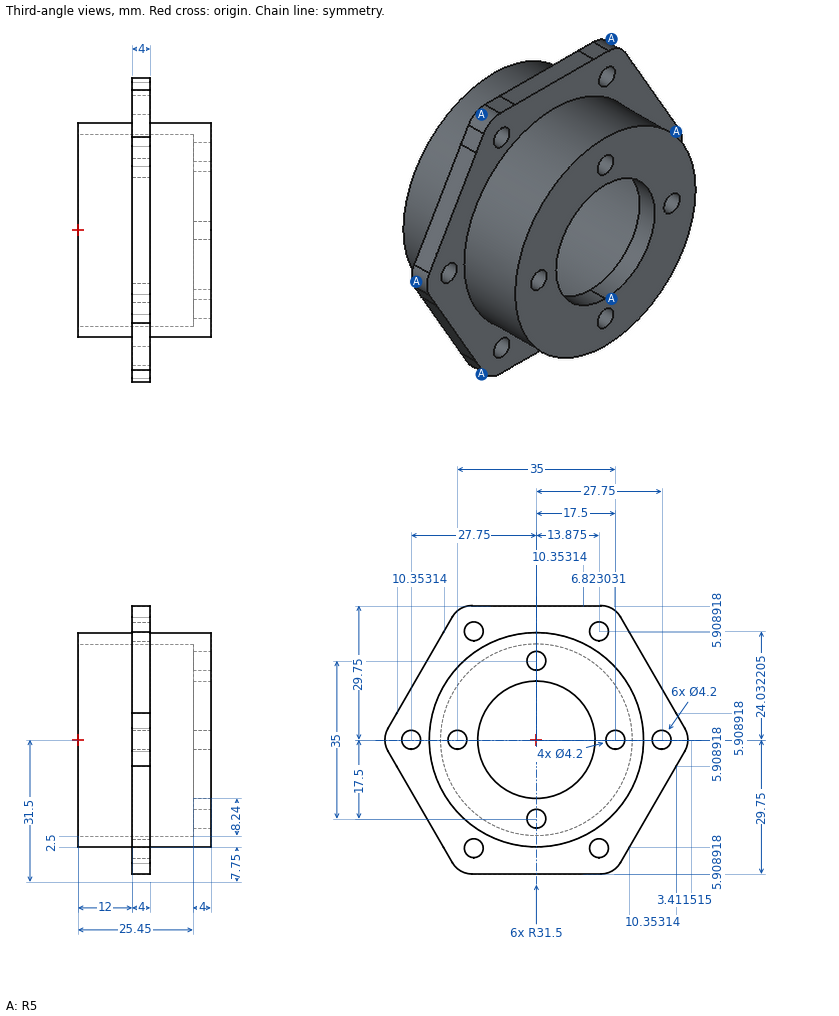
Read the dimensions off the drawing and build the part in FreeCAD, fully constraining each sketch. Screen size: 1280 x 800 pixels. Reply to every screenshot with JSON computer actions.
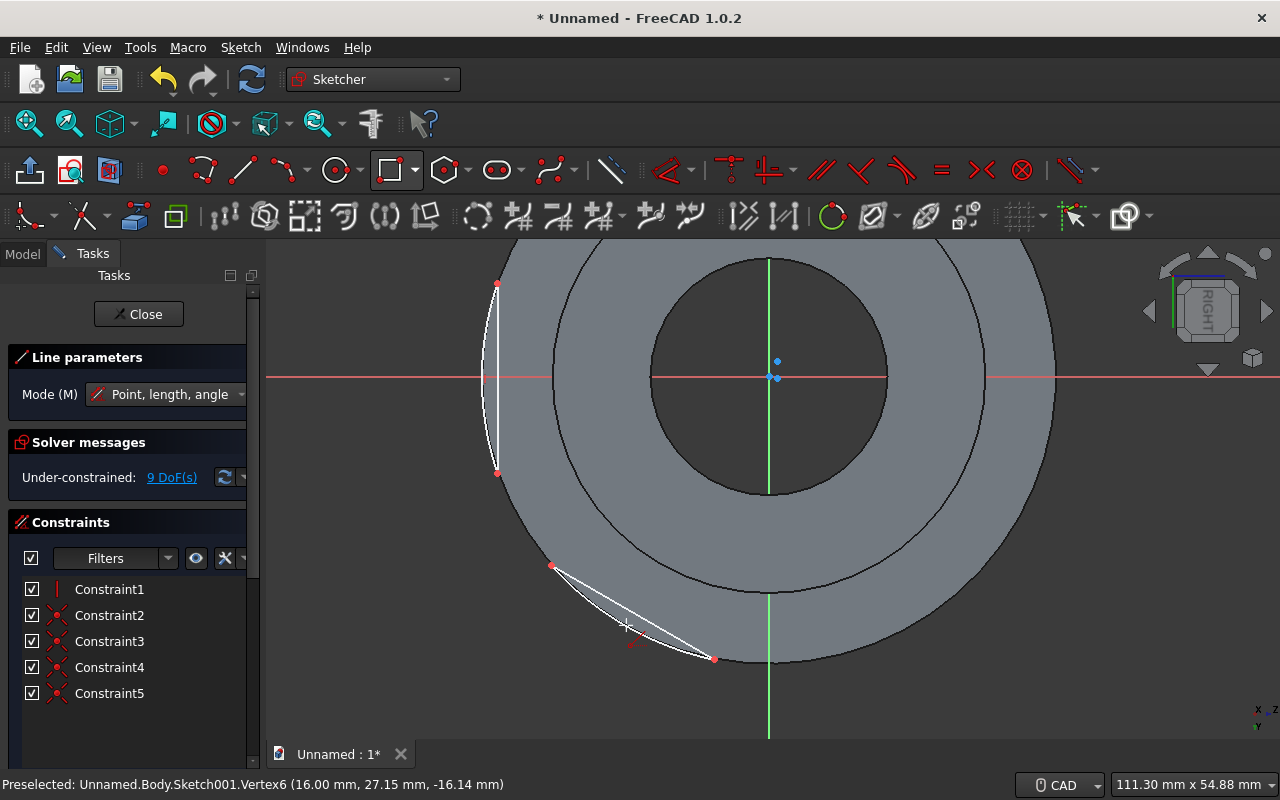
{"action": "left_click", "coordinate": [986, 564]}
{"action": "left_click", "coordinate": [823, 659]}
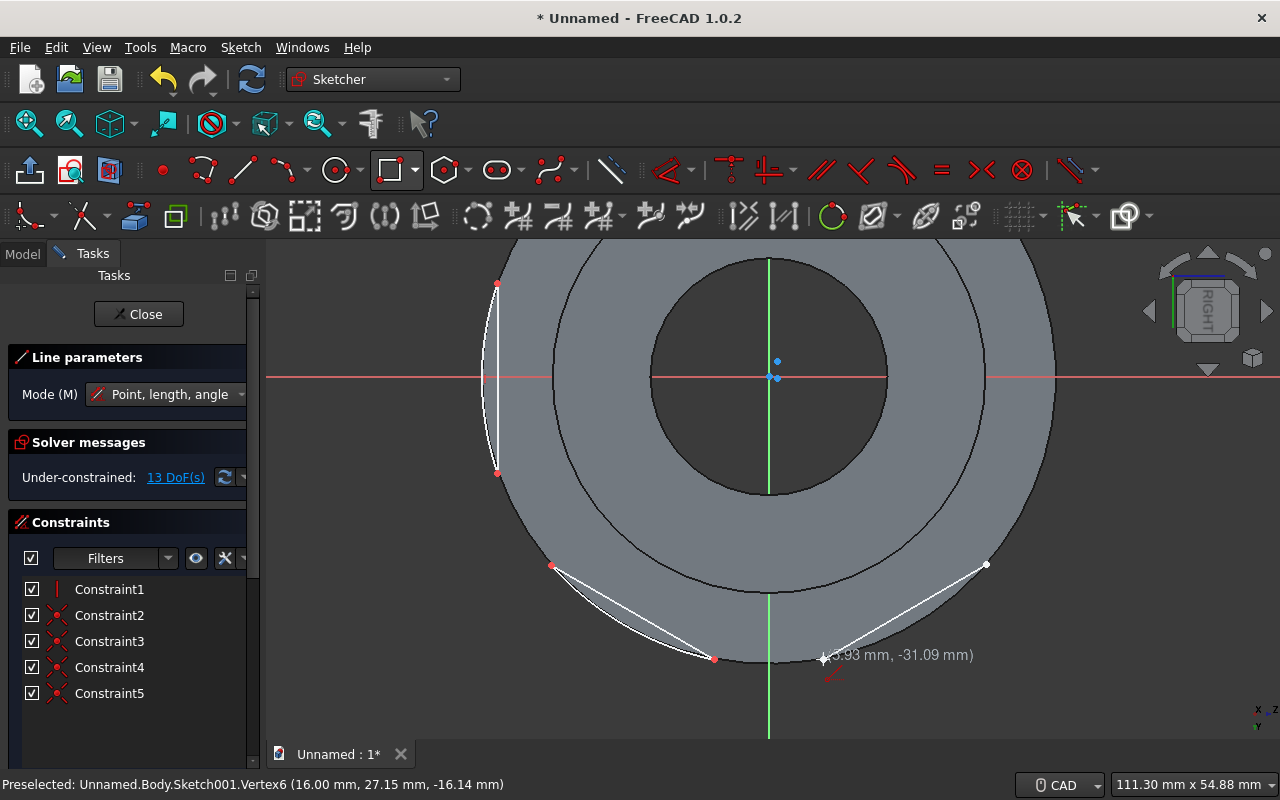
{"action": "left_click", "coordinate": [284, 170]}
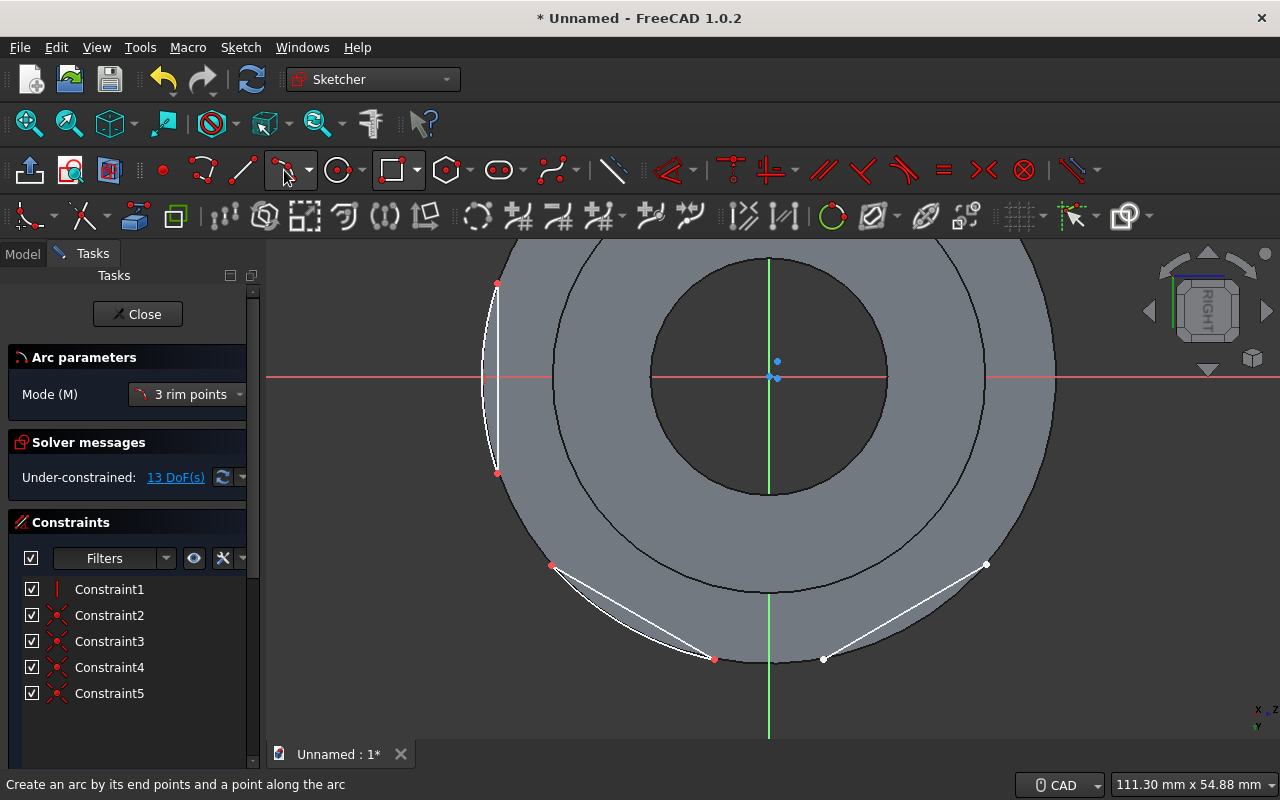
{"action": "left_click", "coordinate": [823, 660]}
{"action": "left_click", "coordinate": [986, 565]}
{"action": "left_click", "coordinate": [913, 625]}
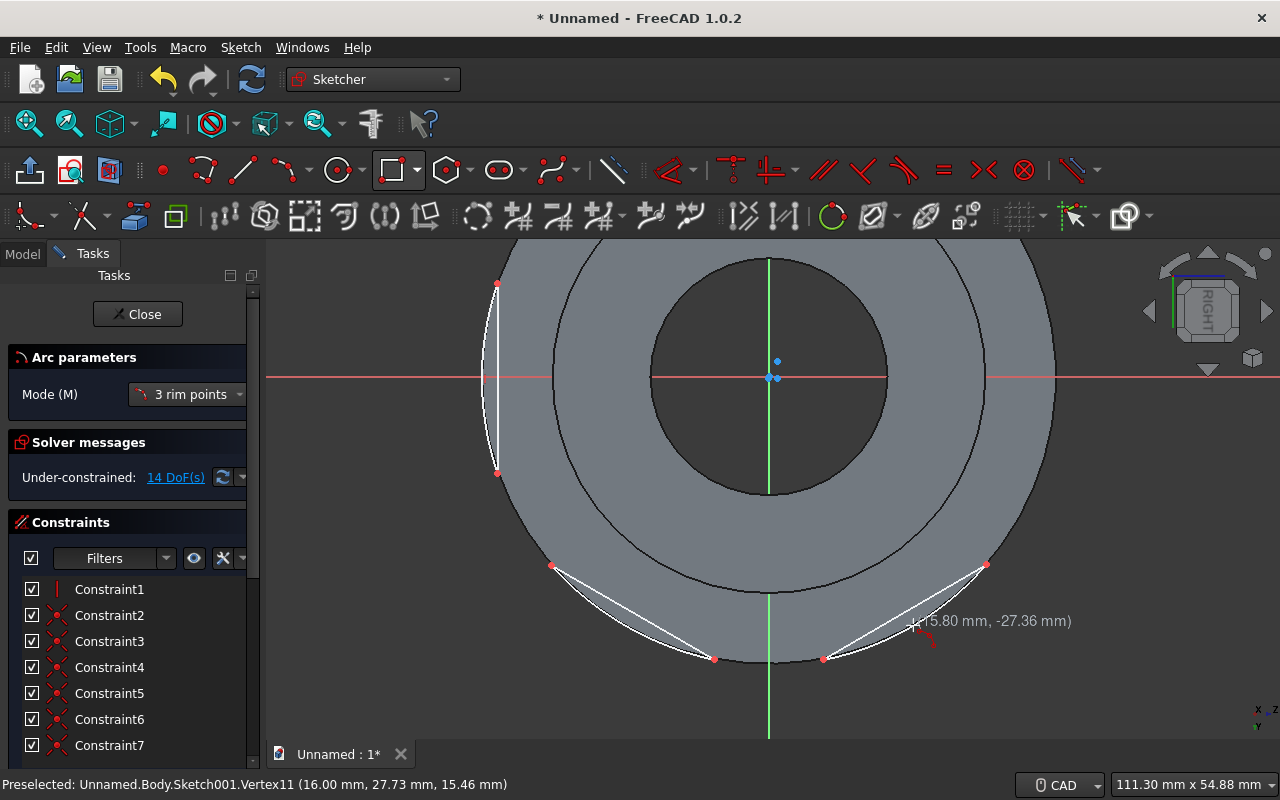
{"action": "key", "text": "g l"}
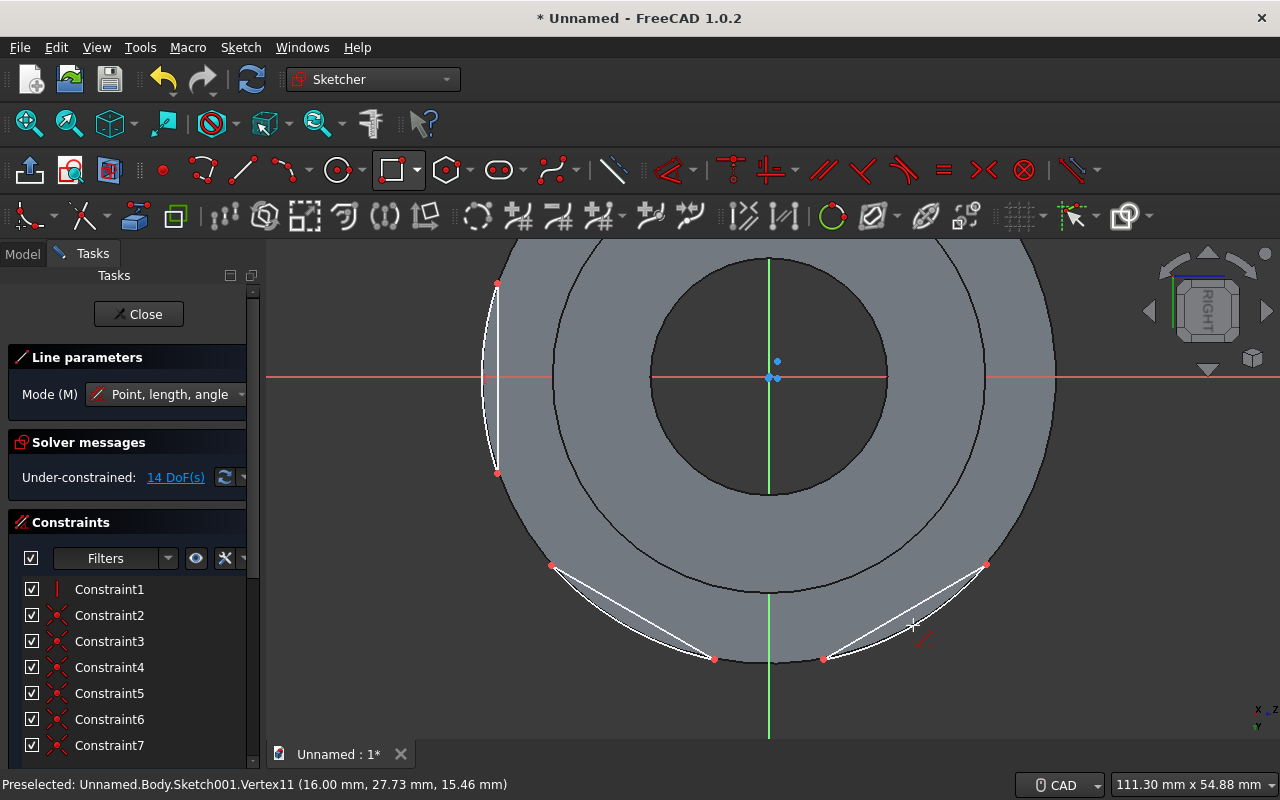
{"action": "left_click", "coordinate": [1040, 282]}
{"action": "left_click", "coordinate": [1040, 471]}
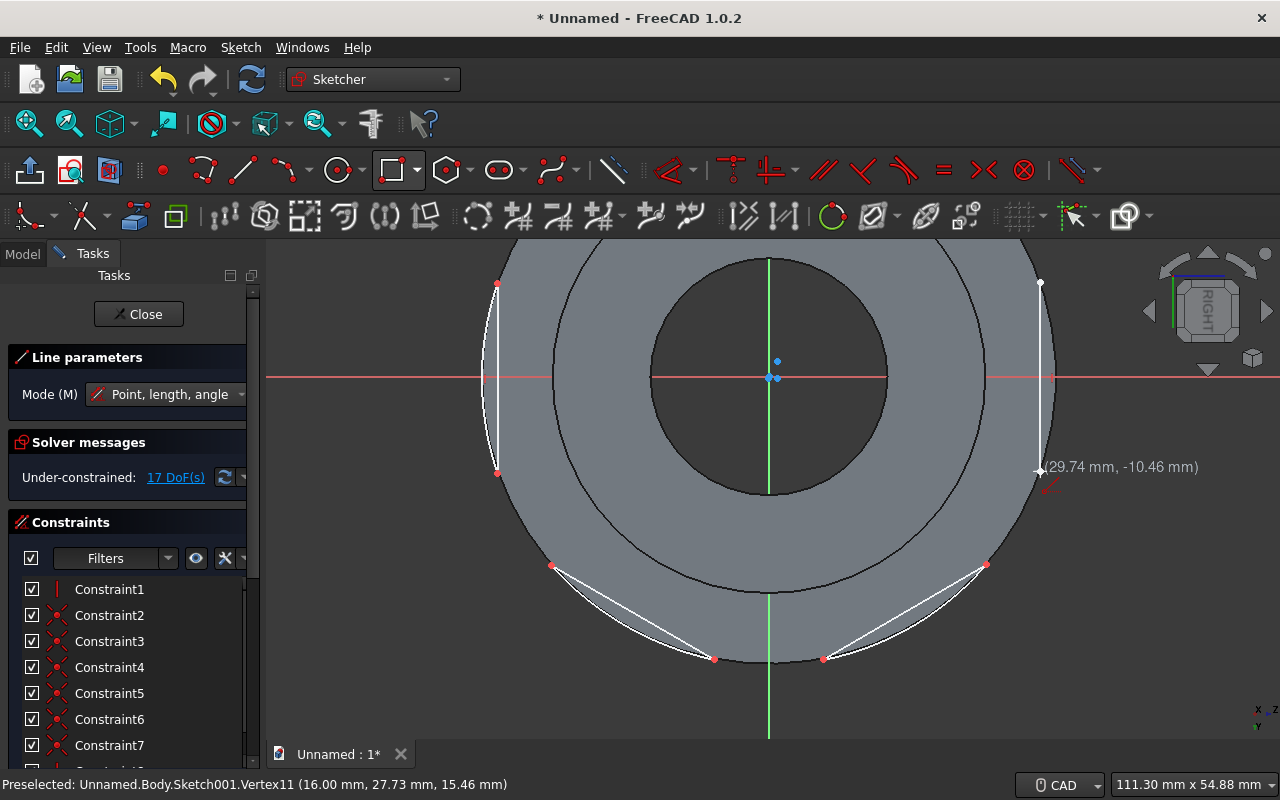
{"action": "left_click", "coordinate": [284, 170]}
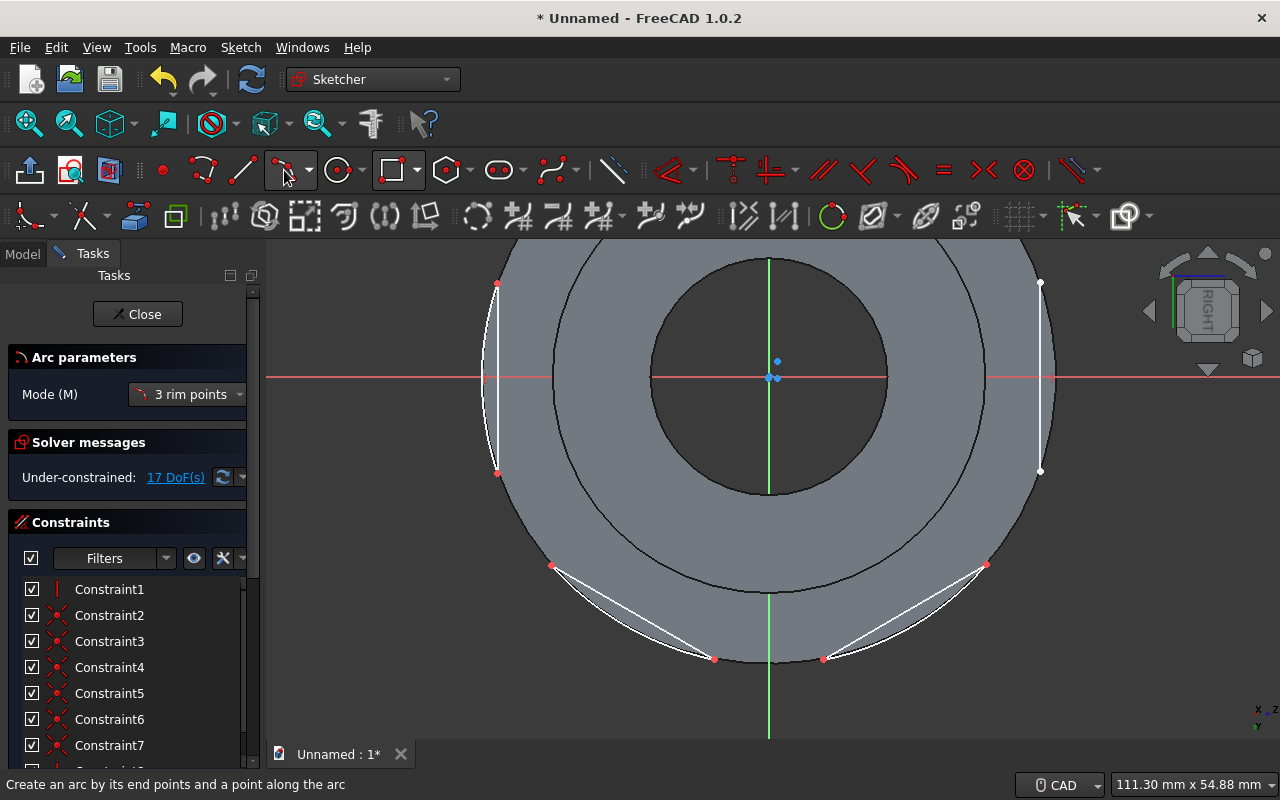
{"action": "left_click", "coordinate": [1040, 472]}
{"action": "left_click", "coordinate": [1040, 283]}
{"action": "left_click", "coordinate": [1055, 396]}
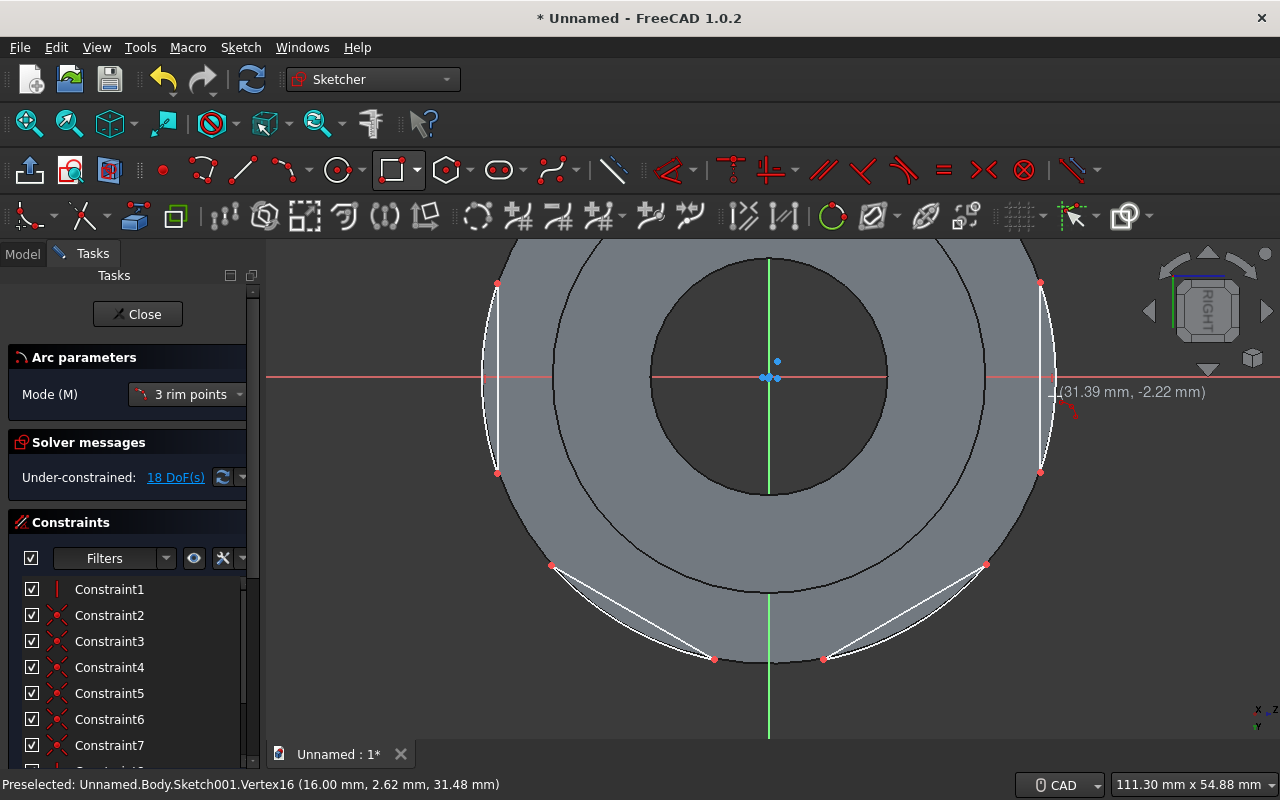
{"action": "key", "text": "g l"}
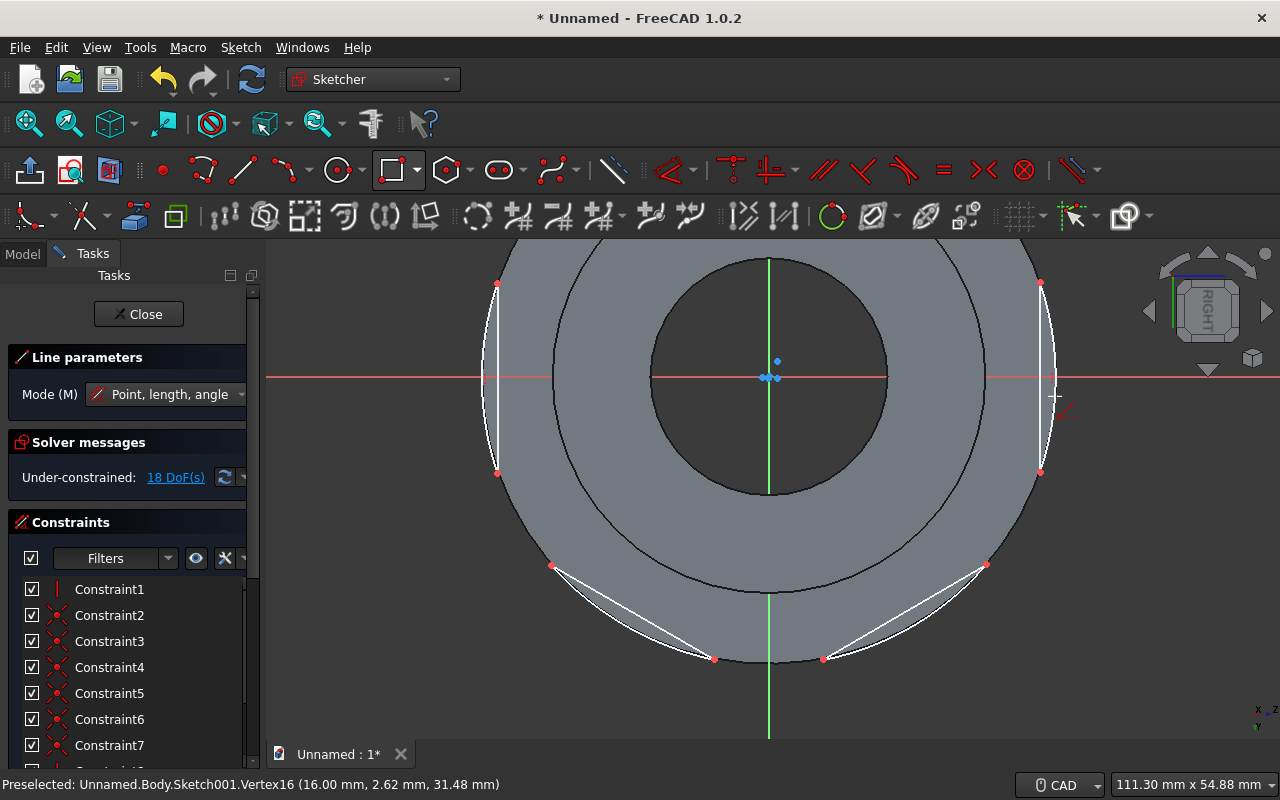
{"action": "scroll", "coordinate": [626, 626], "scroll_direction": "down", "scroll_amount": 3}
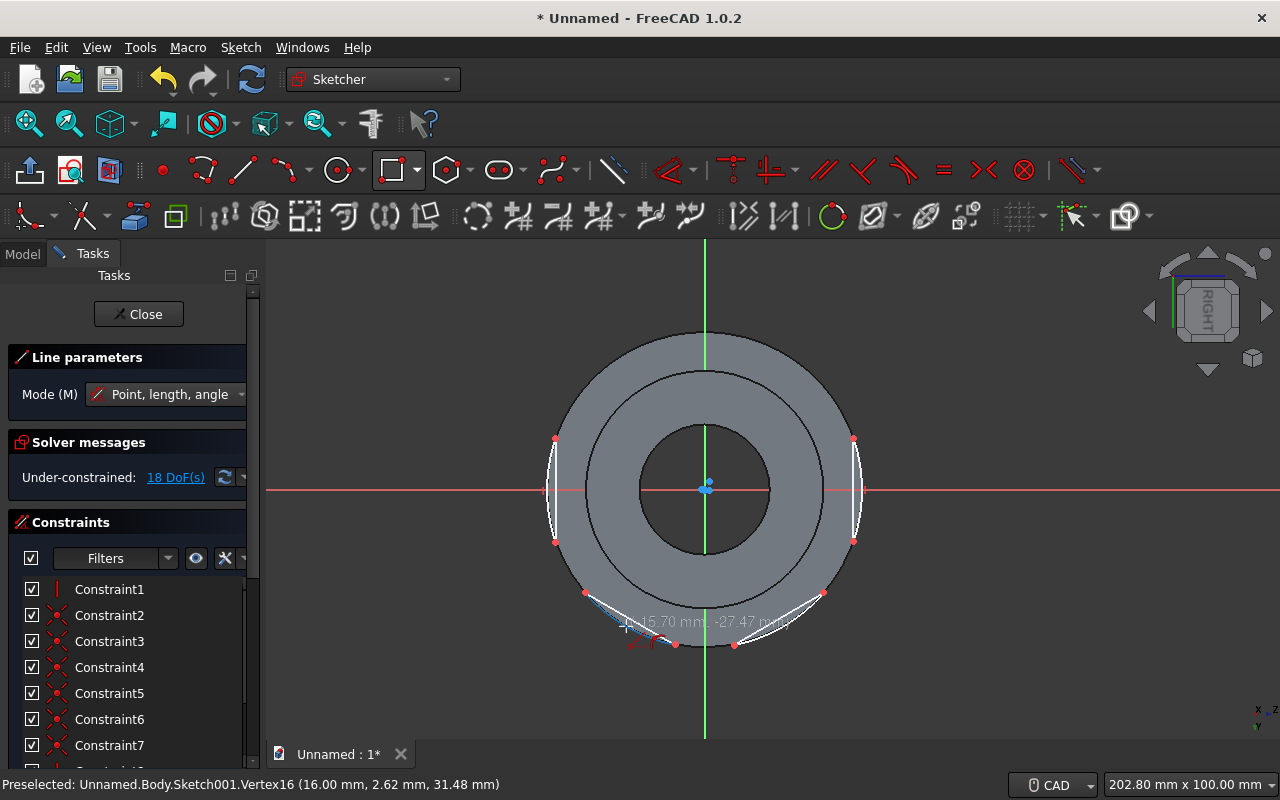
{"action": "left_click", "coordinate": [734, 335]}
{"action": "left_click", "coordinate": [824, 387]}